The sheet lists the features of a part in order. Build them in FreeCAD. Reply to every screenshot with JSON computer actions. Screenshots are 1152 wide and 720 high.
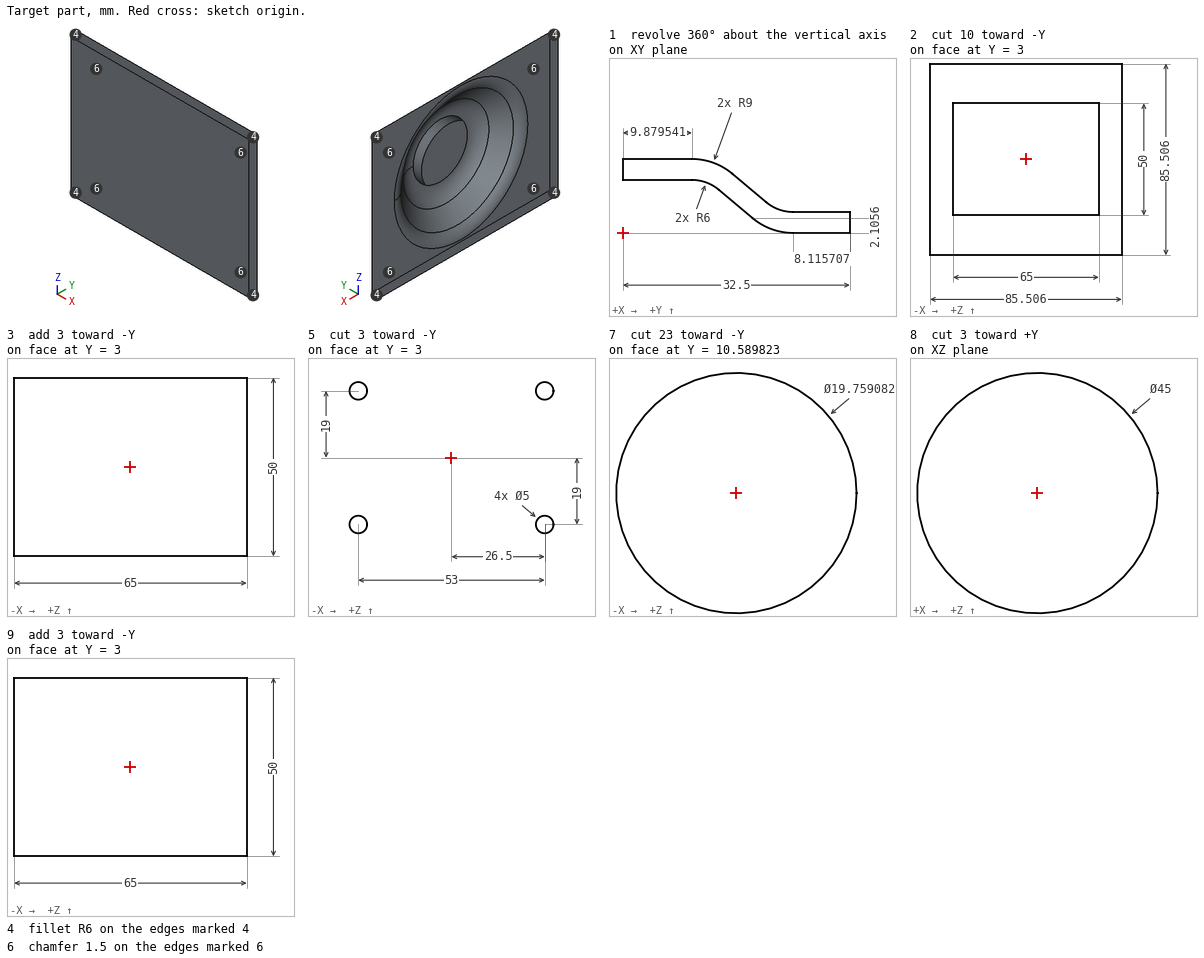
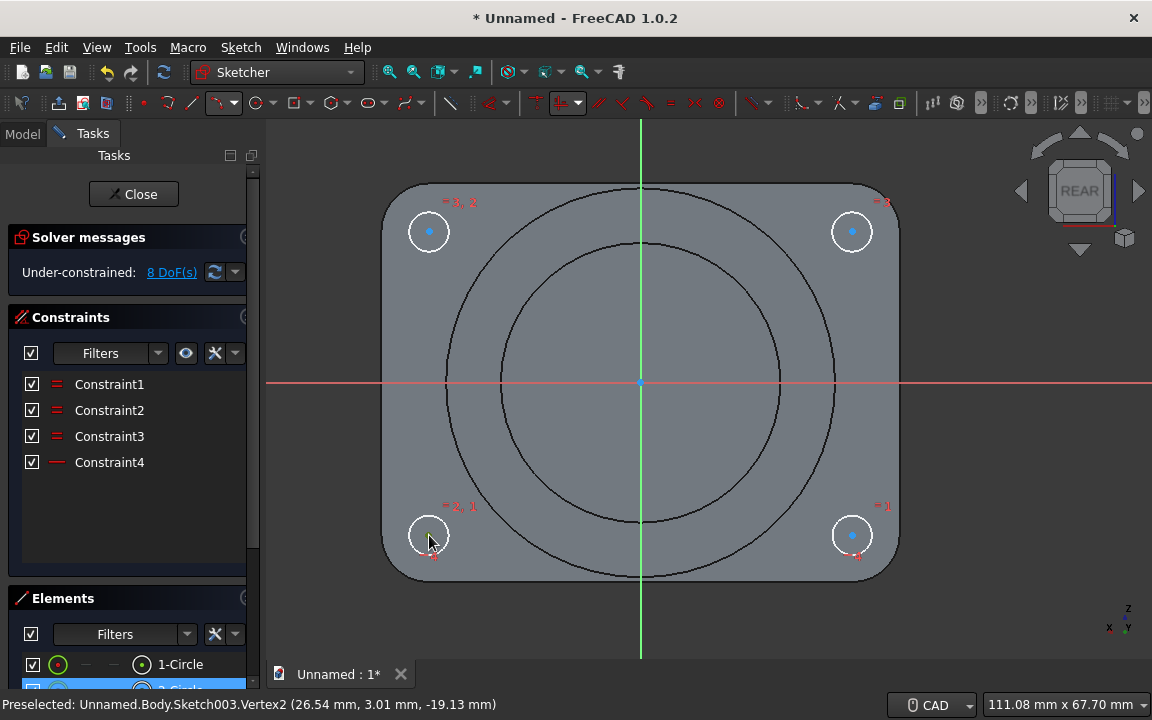
{"action": "left_click", "coordinate": [429, 232]}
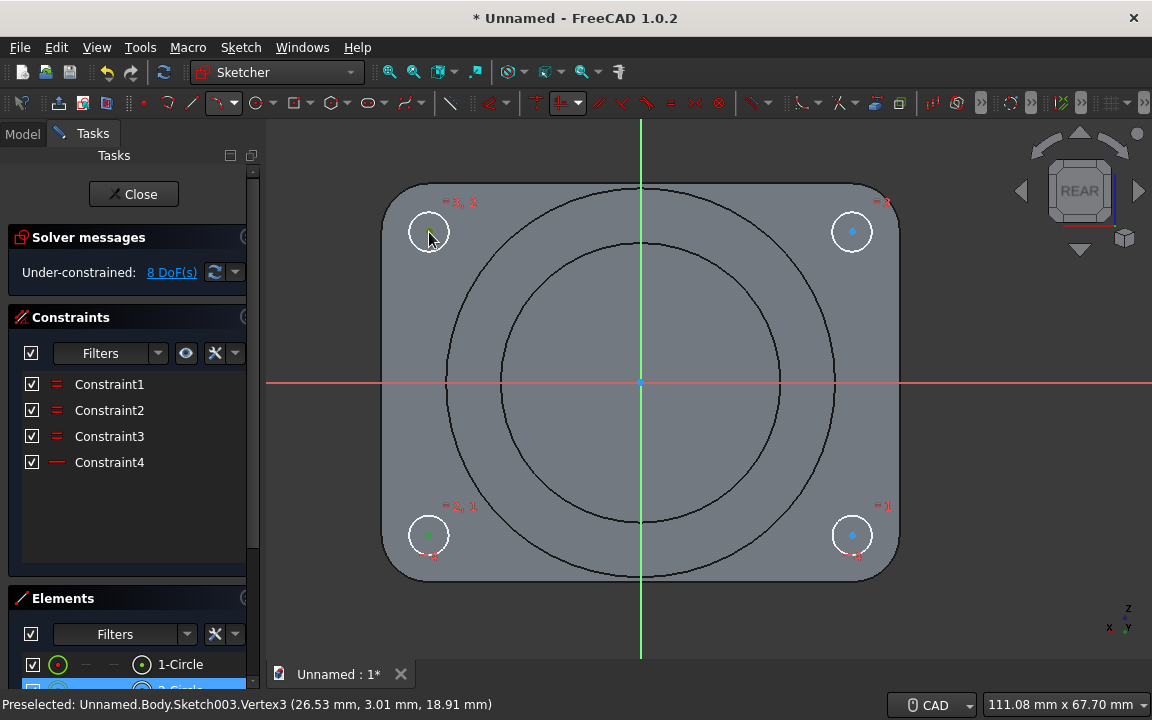
{"action": "left_click", "coordinate": [580, 104]}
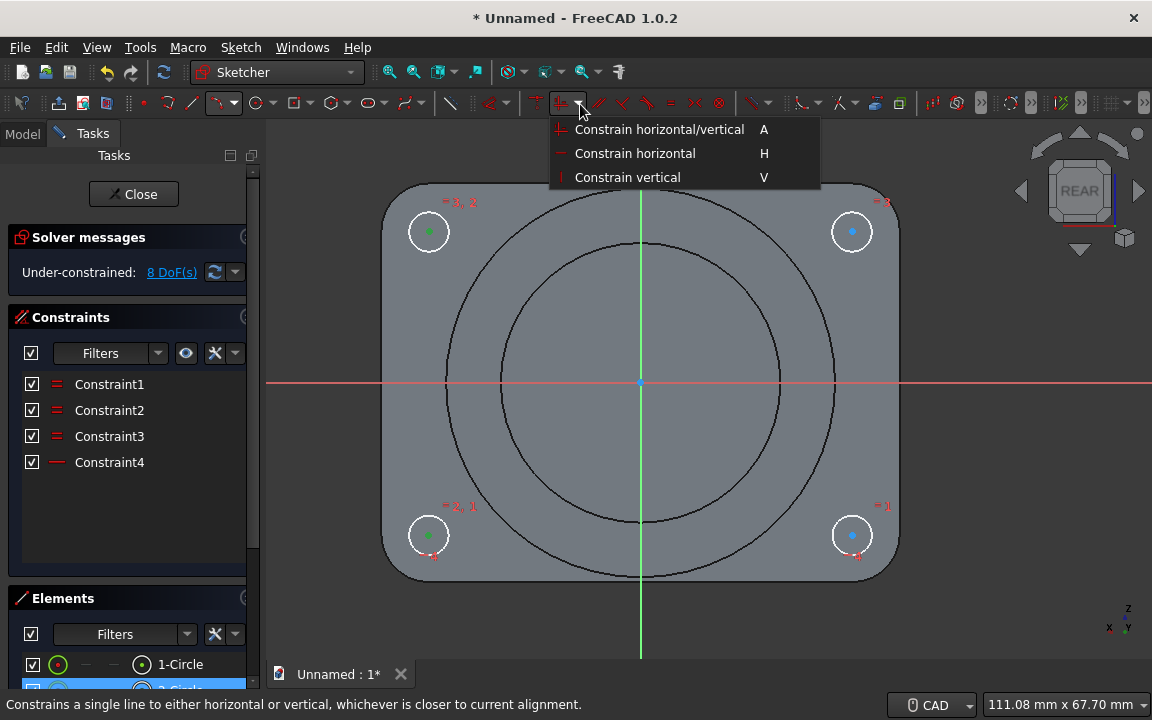
{"action": "left_click", "coordinate": [685, 177]}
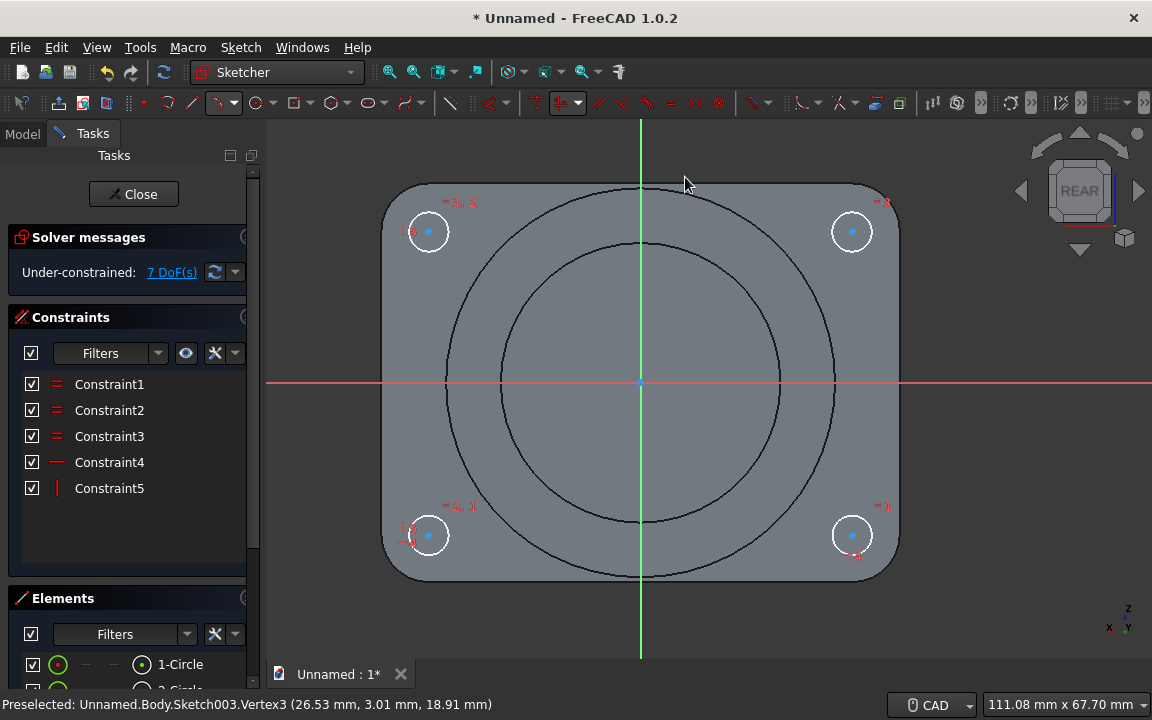
{"action": "left_click", "coordinate": [852, 535]}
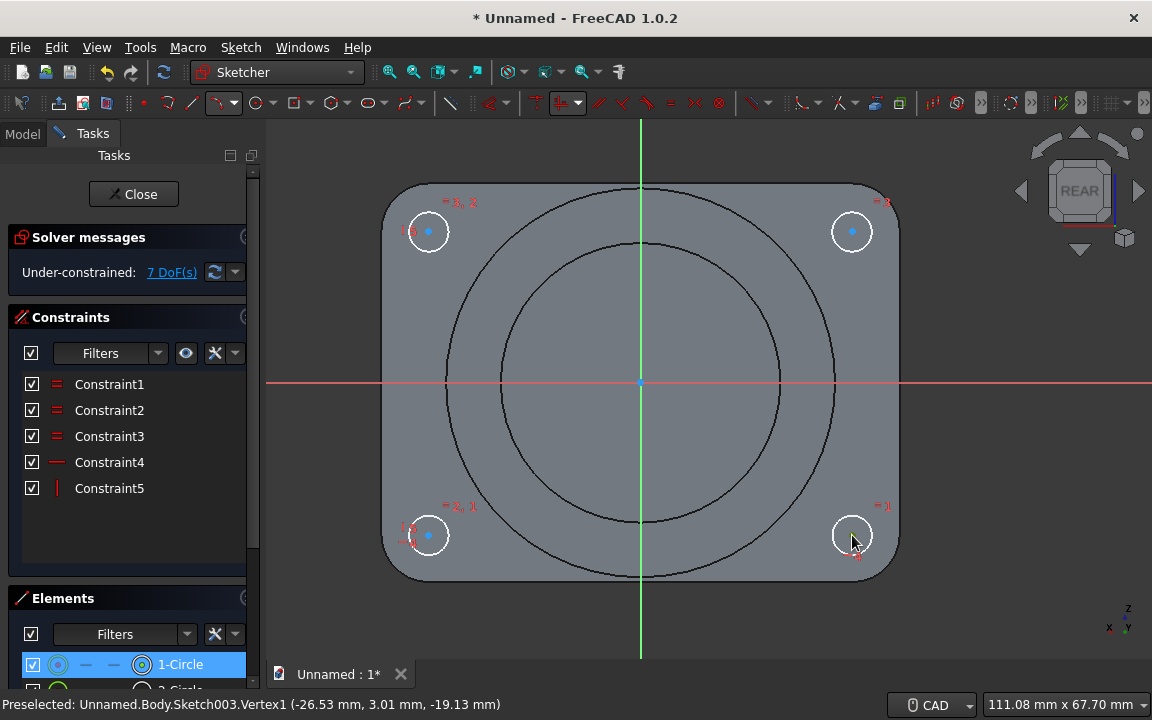
{"action": "left_click", "coordinate": [852, 232]}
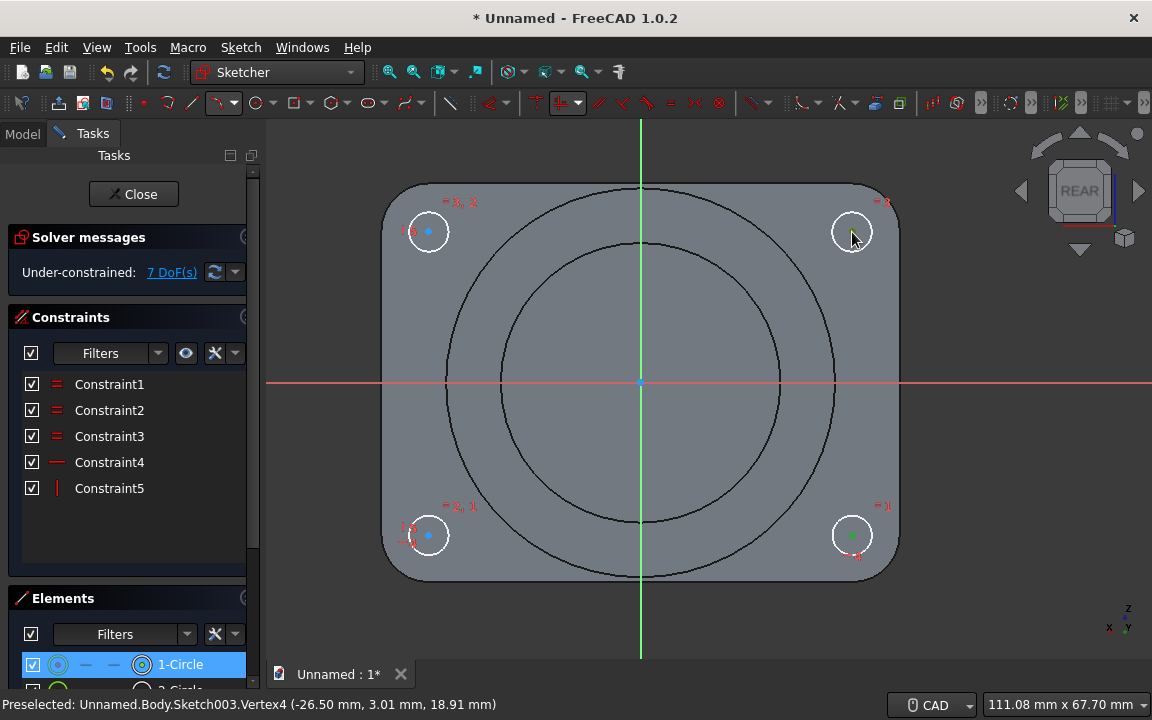
{"action": "key", "text": "v"}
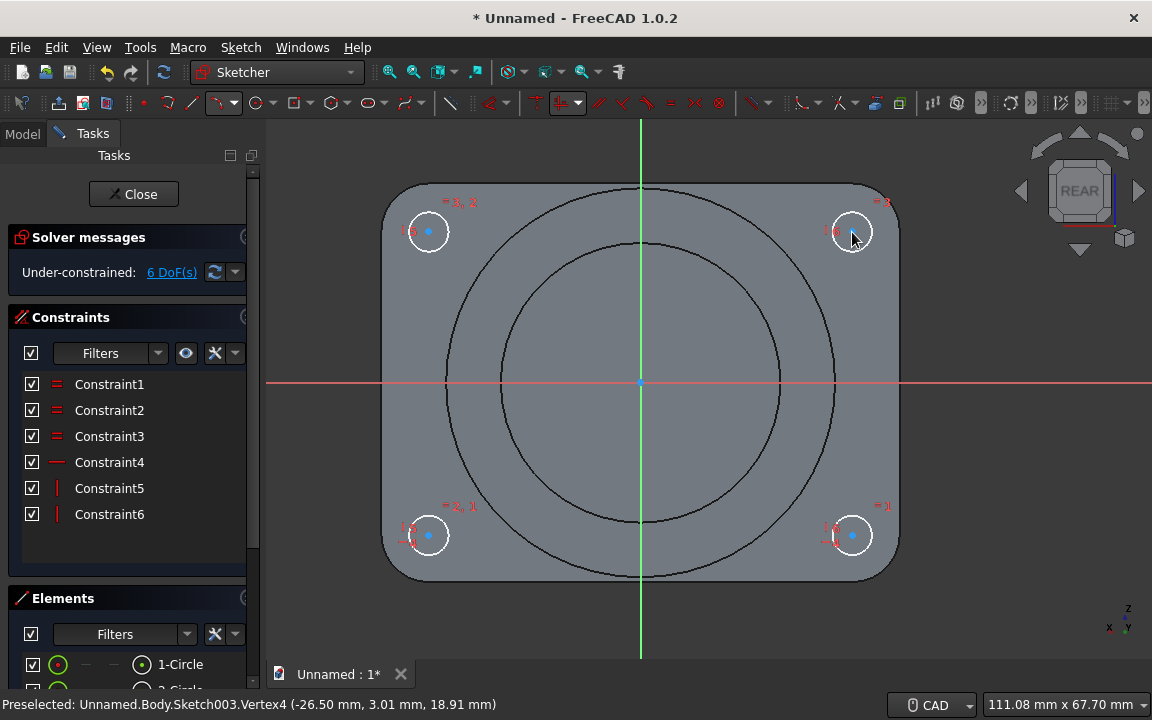
{"action": "left_click", "coordinate": [429, 232]}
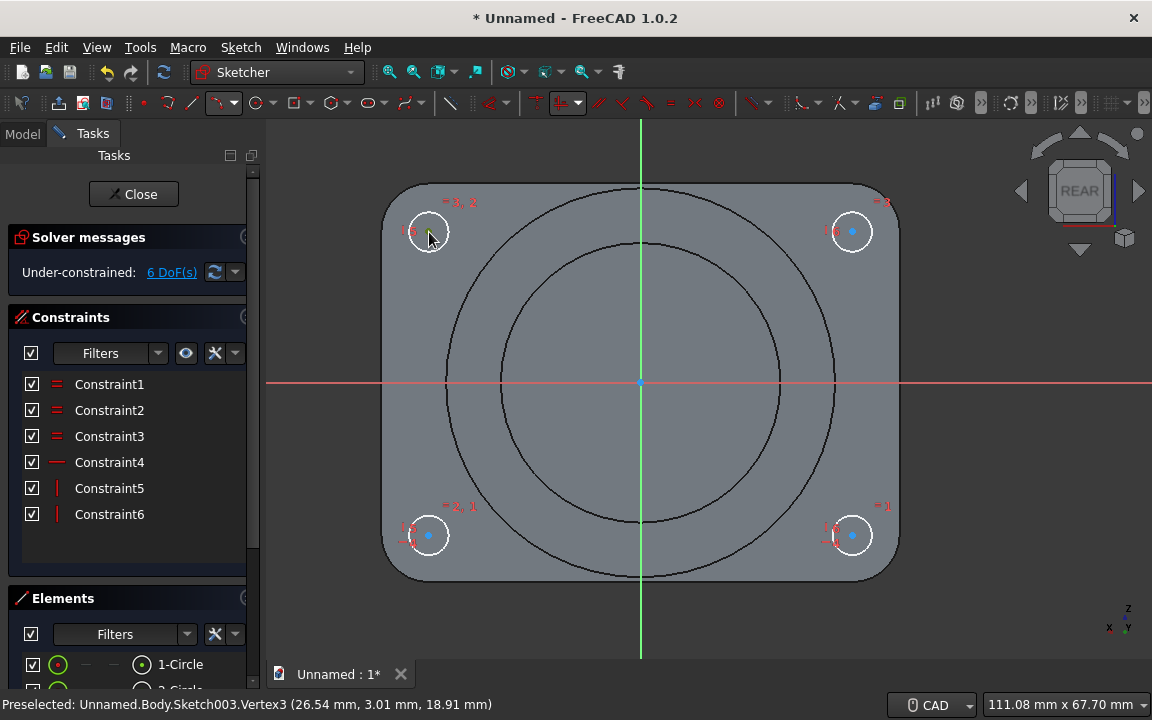
{"action": "left_click", "coordinate": [852, 232]}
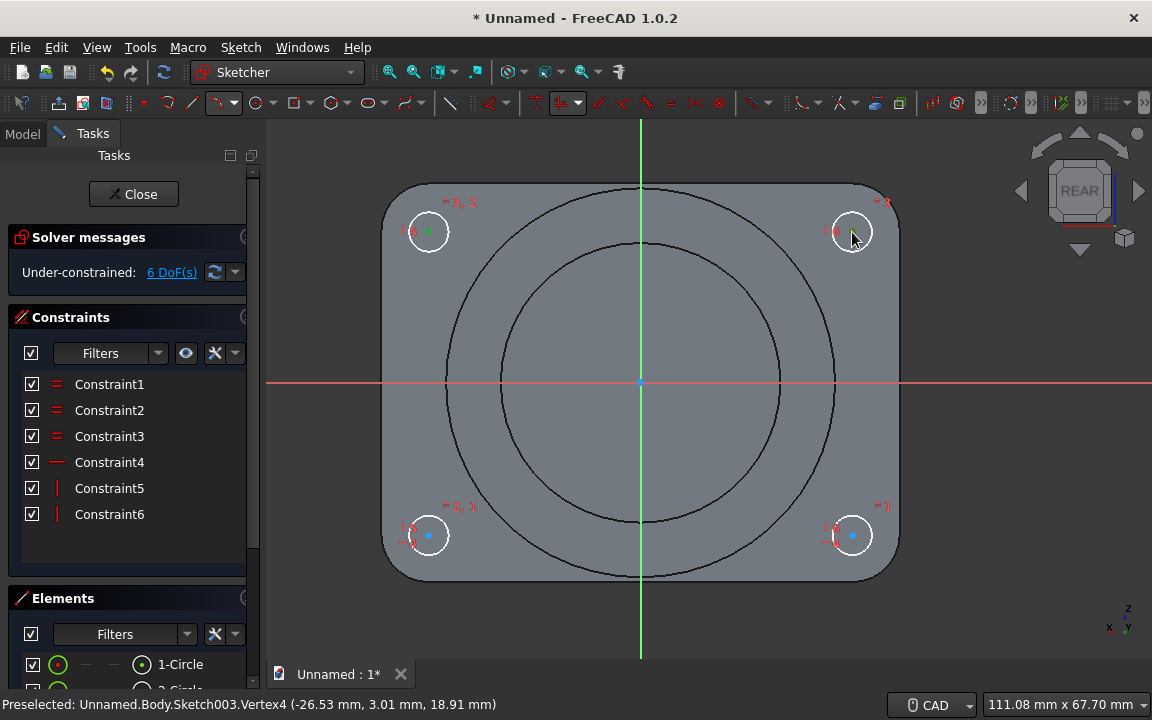
{"action": "key", "text": "h"}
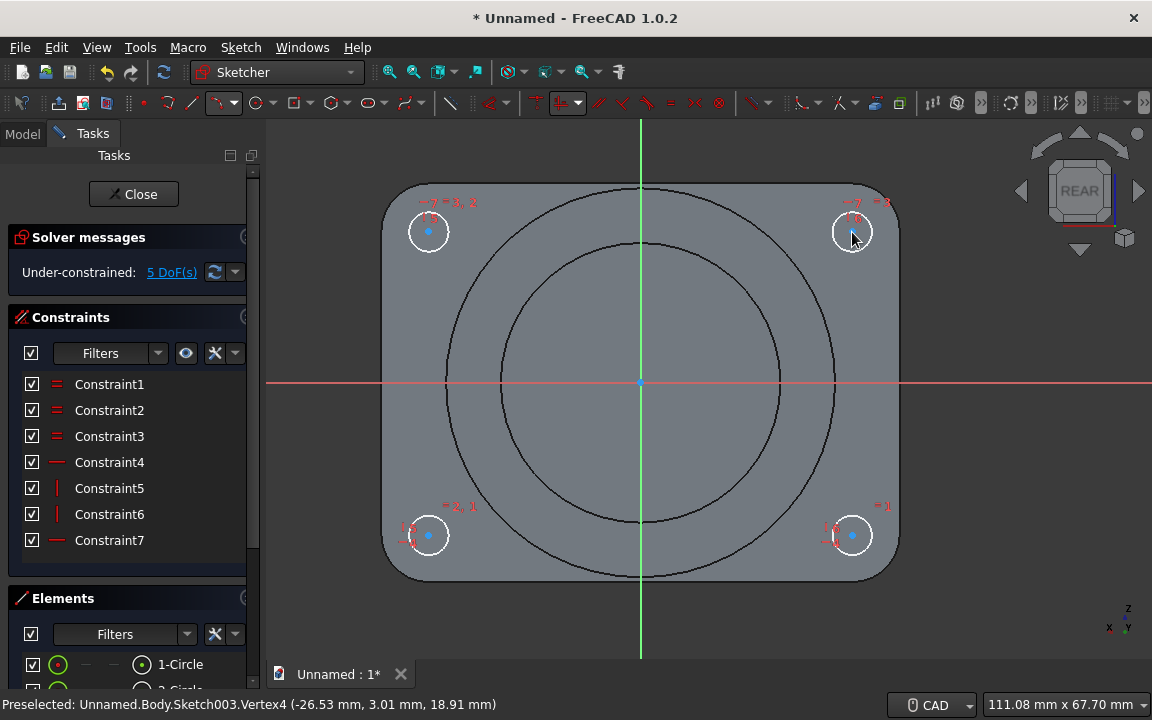
{"action": "left_click", "coordinate": [490, 104]}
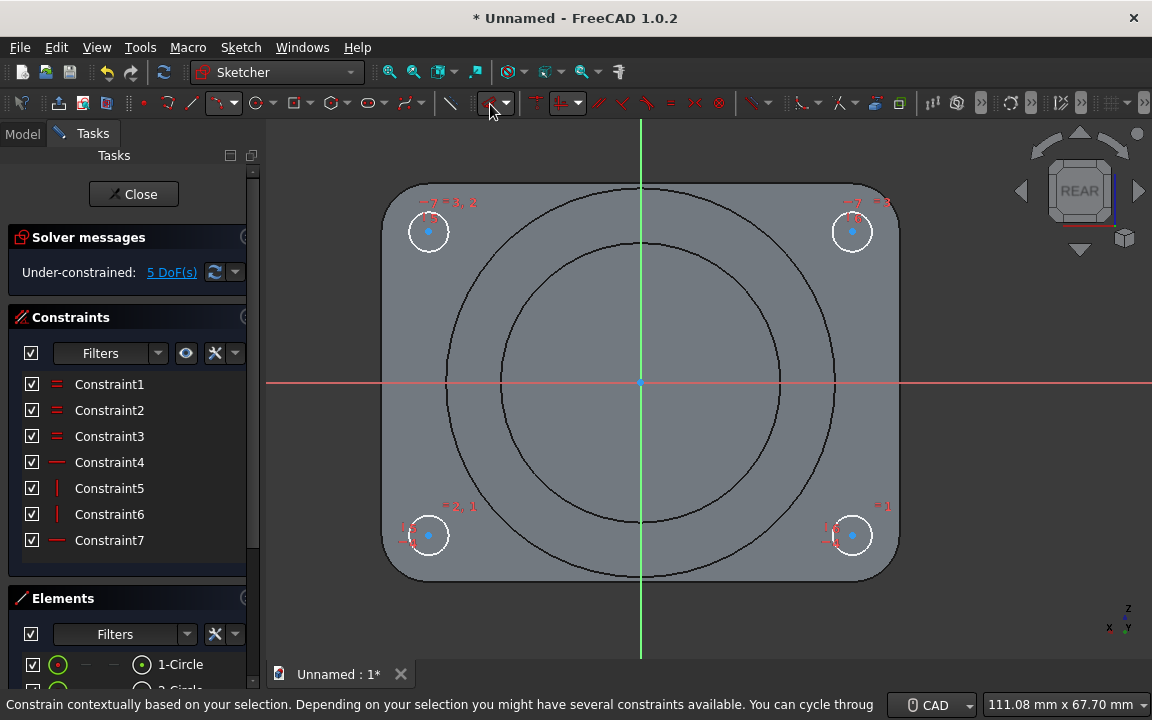
{"action": "left_click", "coordinate": [866, 521]}
{"action": "left_click", "coordinate": [888, 498]}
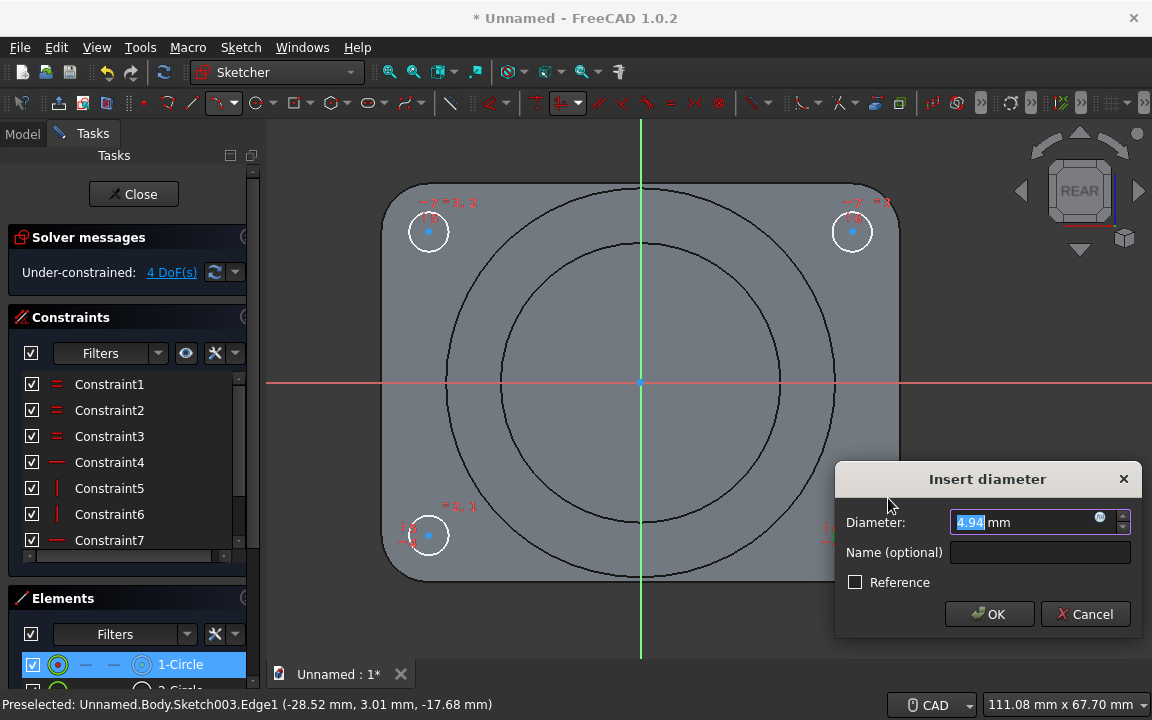
{"action": "type", "text": "5"}
{"action": "key", "text": "Return"}